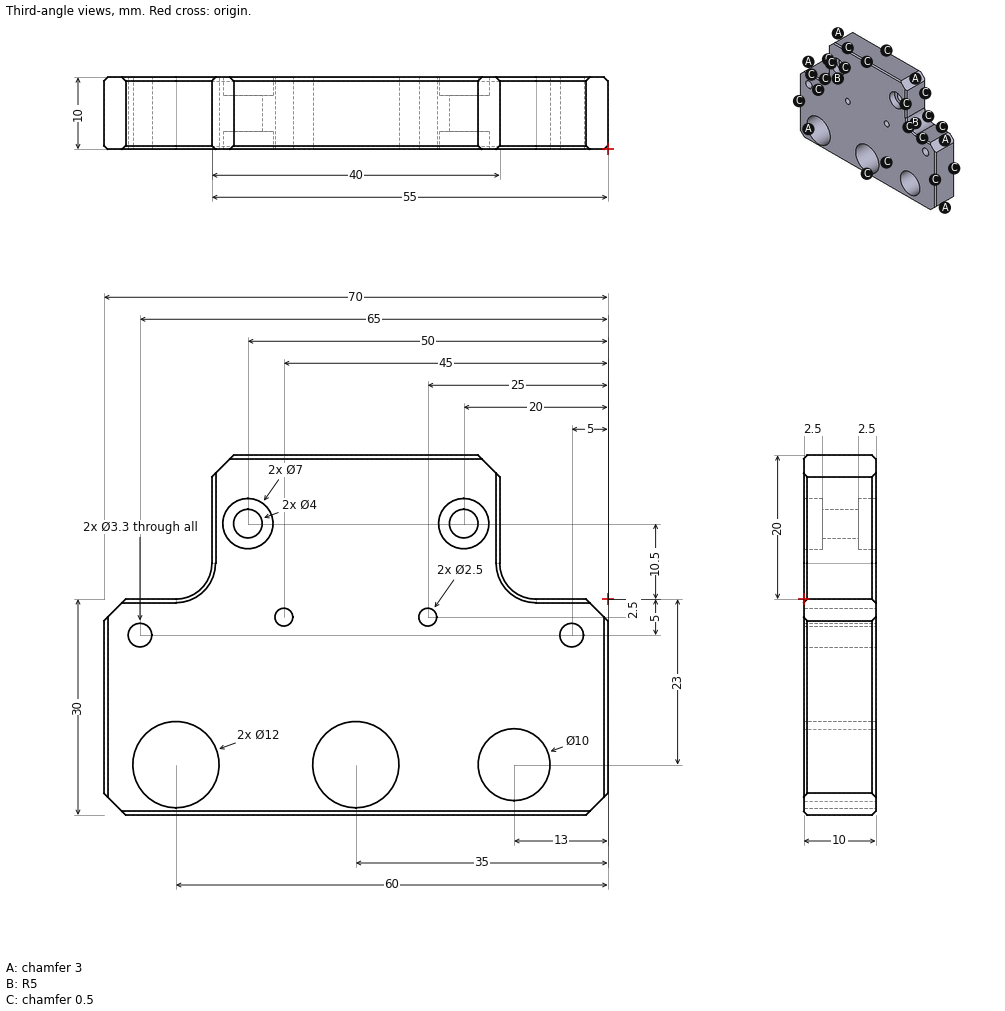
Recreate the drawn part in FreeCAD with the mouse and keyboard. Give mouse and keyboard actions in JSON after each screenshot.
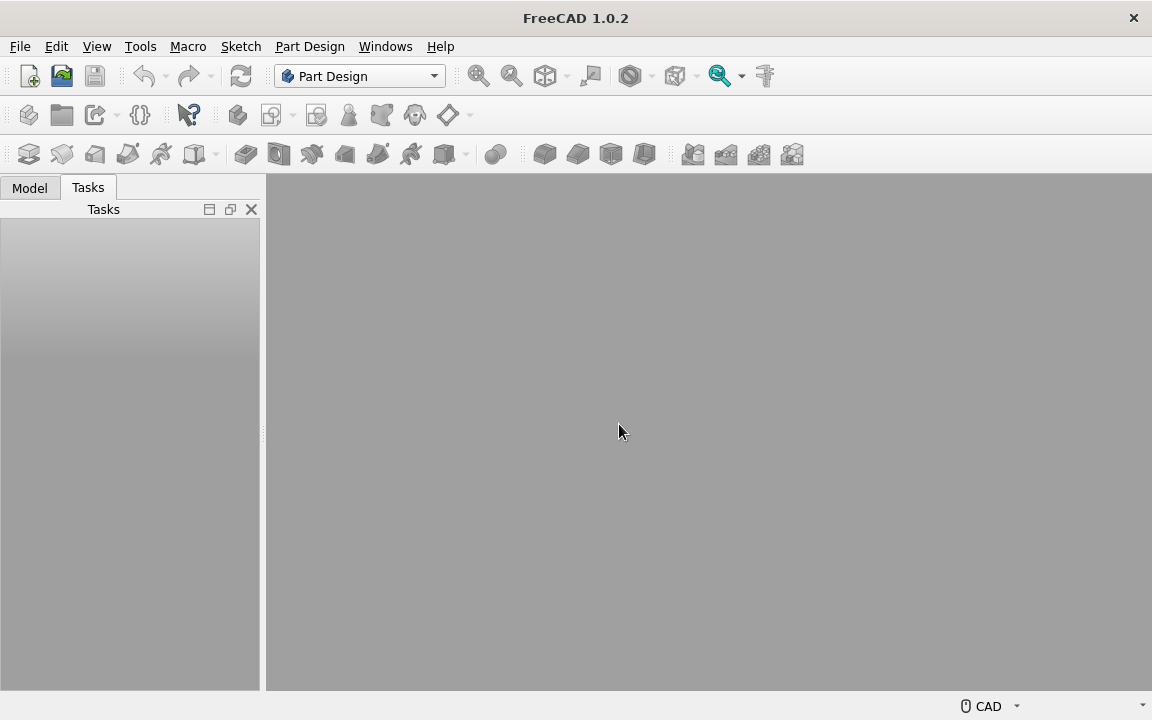
{"action": "left_click", "coordinate": [29, 76]}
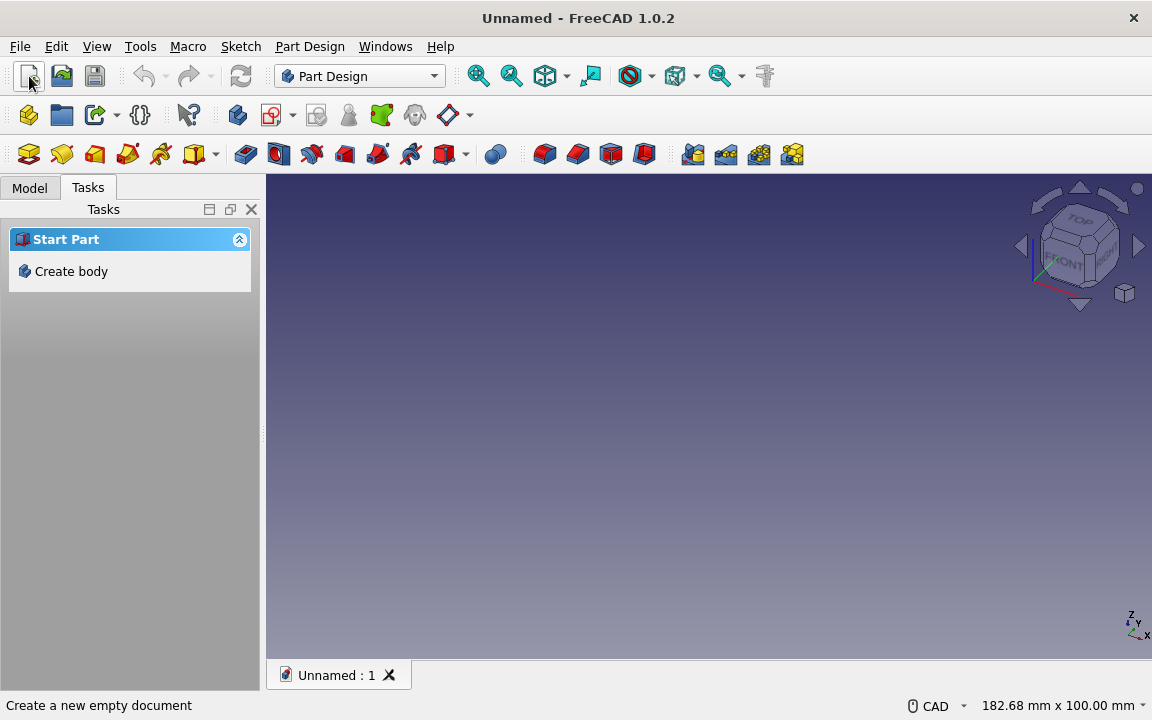
{"action": "left_click", "coordinate": [270, 116]}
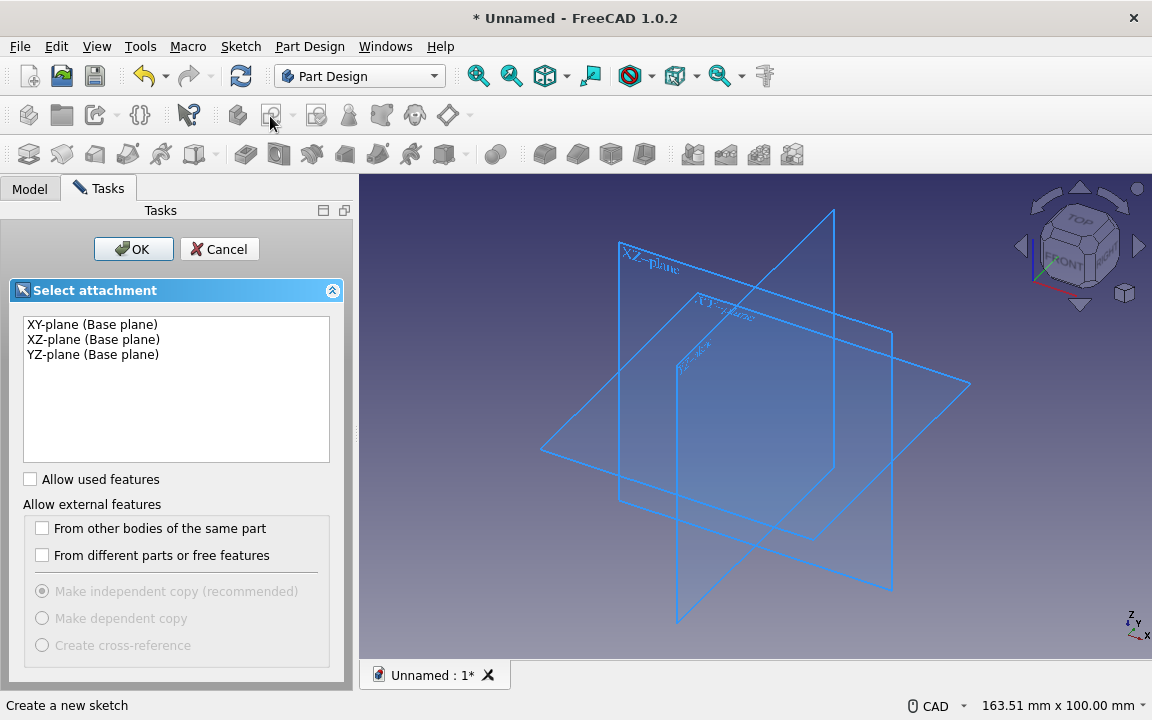
{"action": "left_click", "coordinate": [84, 340]}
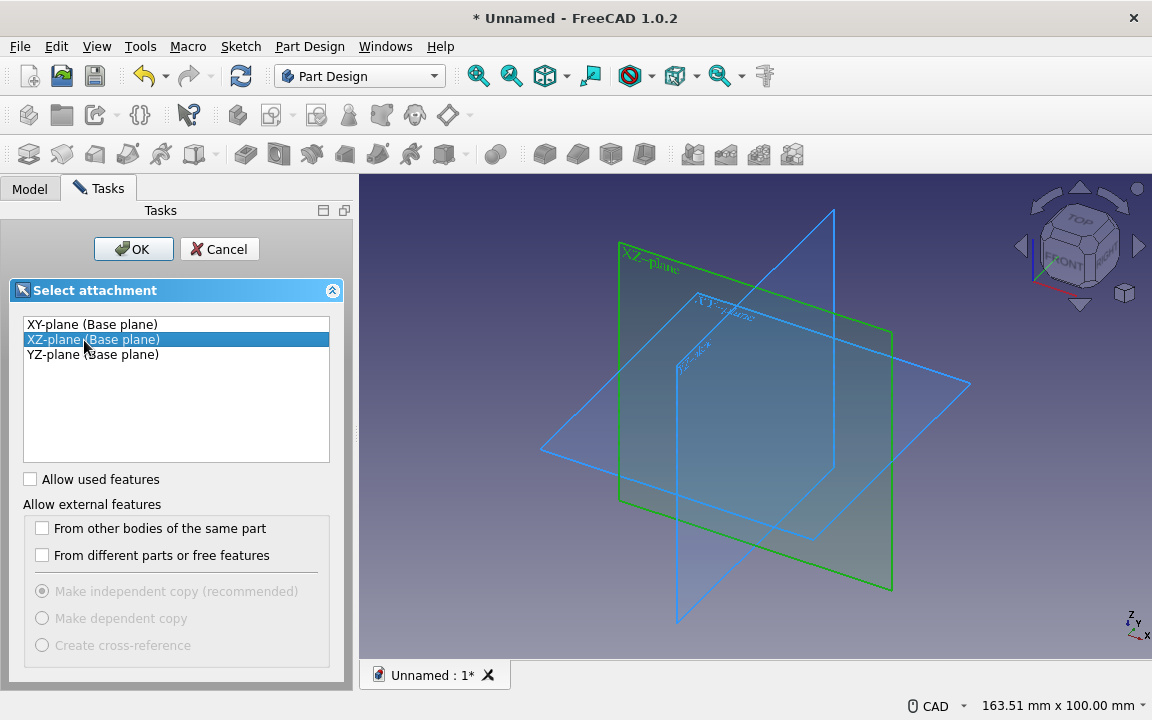
{"action": "left_click", "coordinate": [134, 249]}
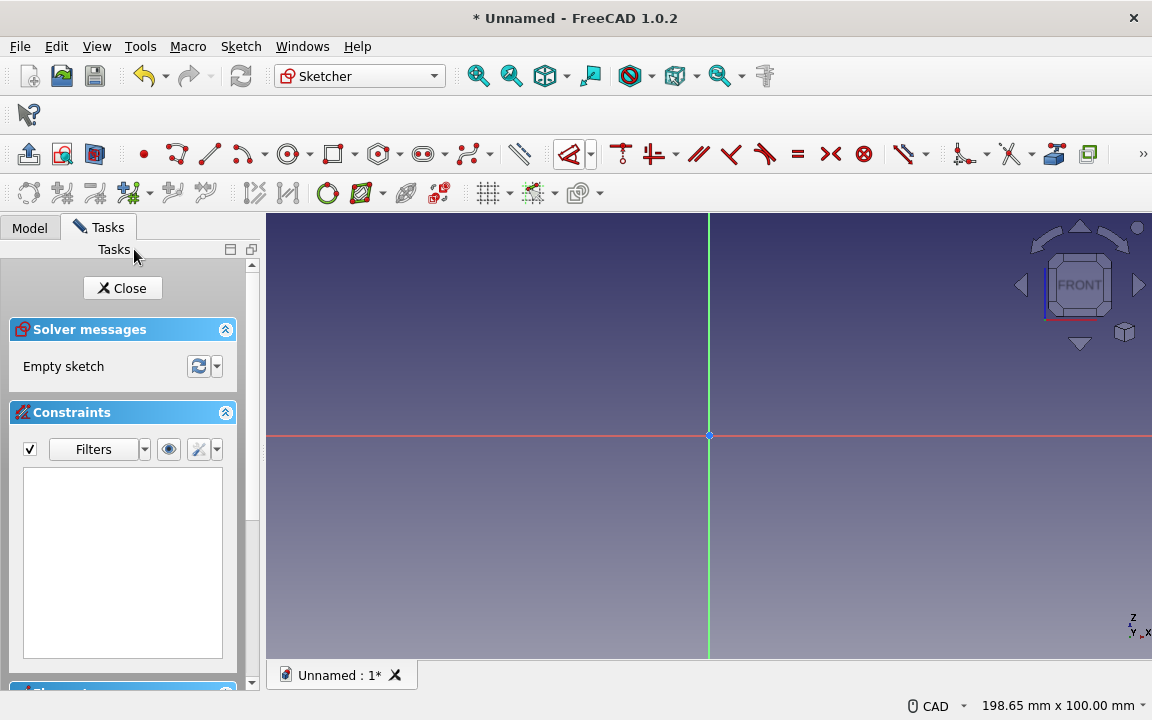
{"action": "scroll", "coordinate": [375, 631], "scroll_direction": "up", "scroll_amount": 2}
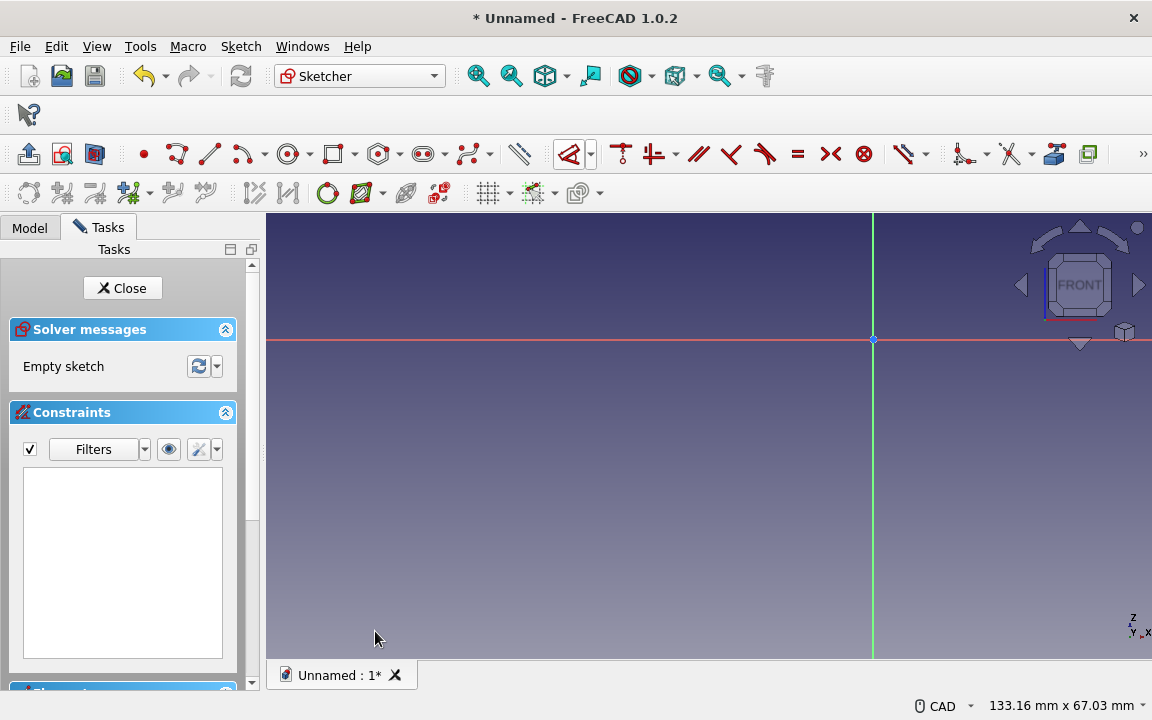
{"action": "left_click", "coordinate": [332, 154]}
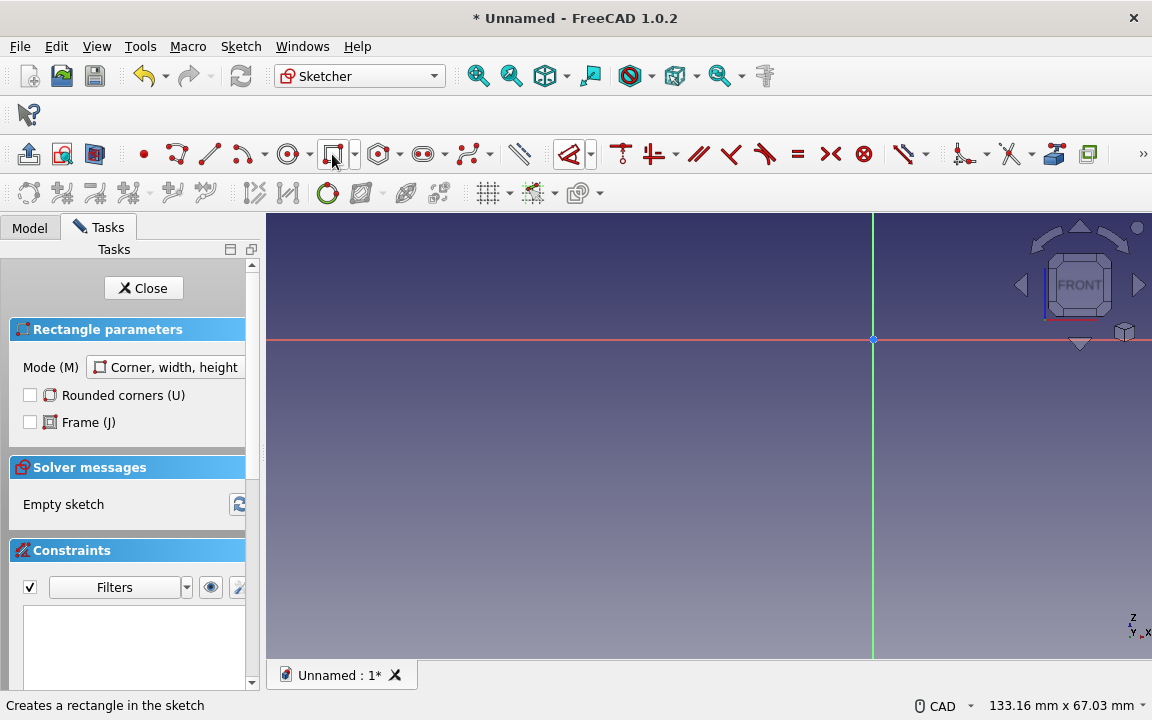
{"action": "left_click", "coordinate": [873, 340]}
{"action": "left_click", "coordinate": [407, 539]}
{"action": "key", "text": "Escape"}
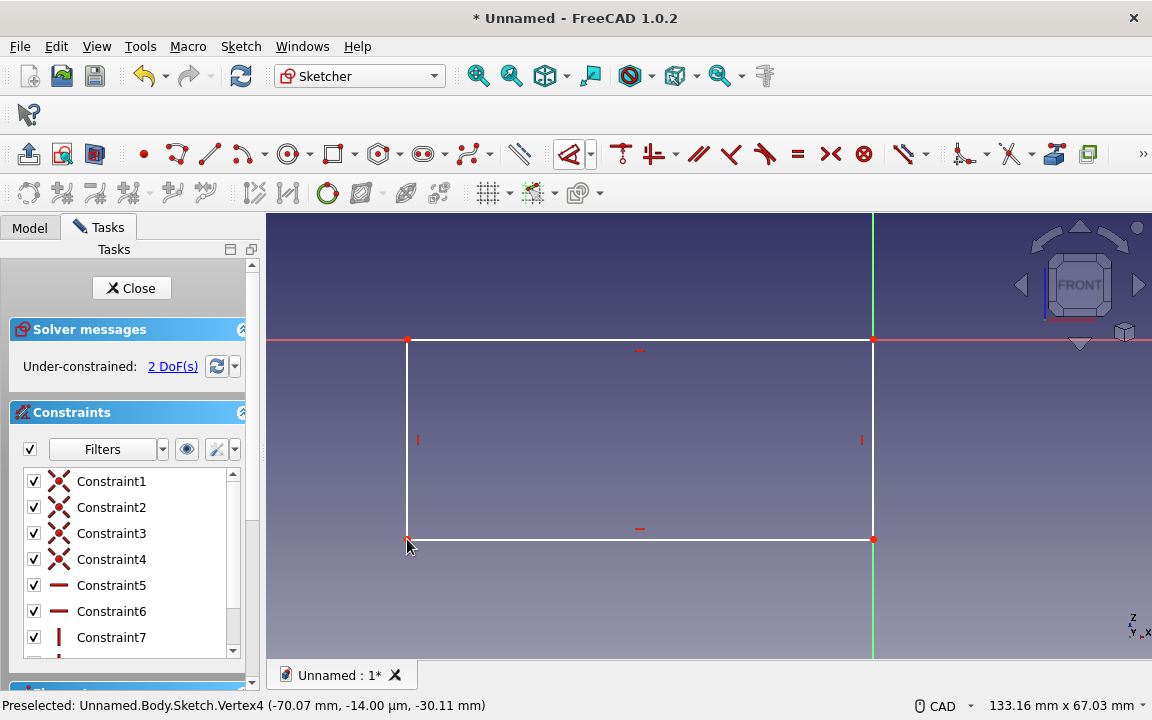
{"action": "left_click", "coordinate": [733, 340]}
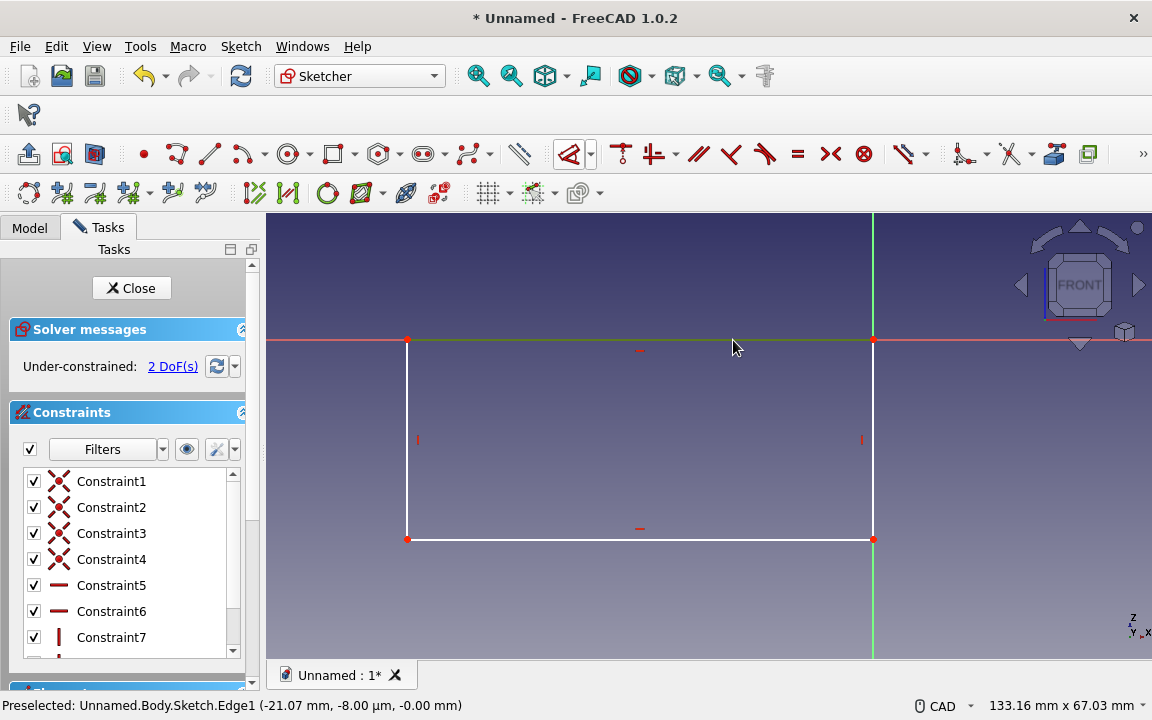
{"action": "key", "text": "l"}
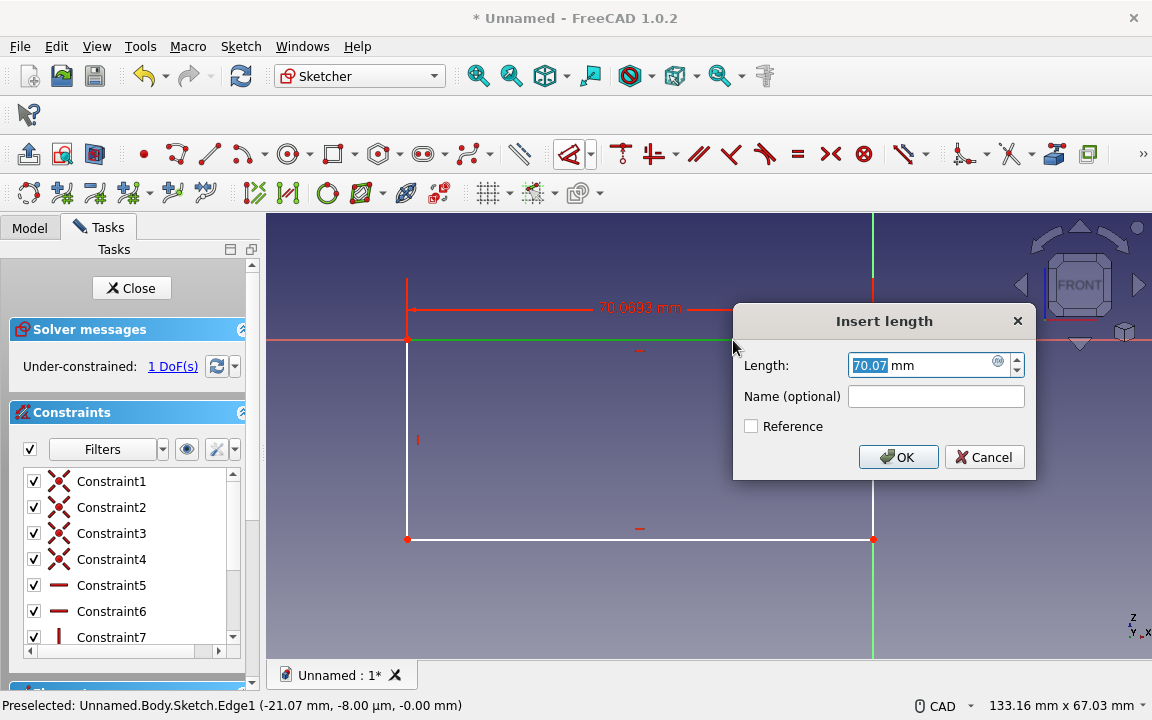
{"action": "type", "text": "70"}
{"action": "key", "text": "Return"}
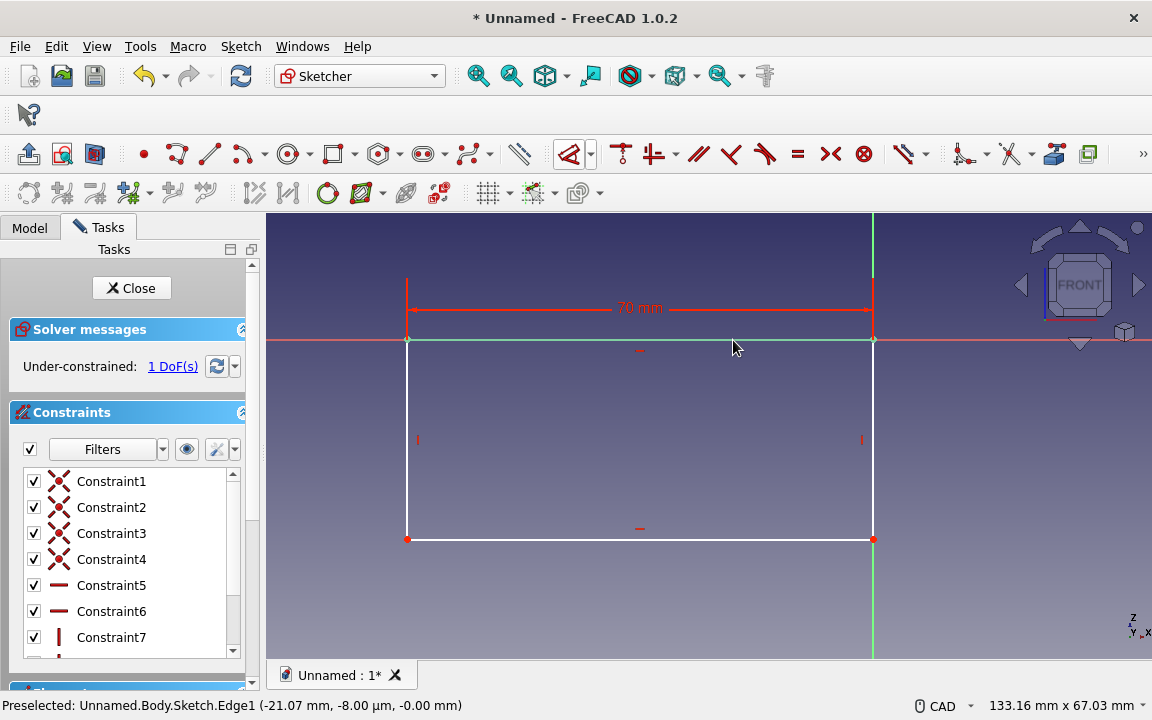
{"action": "left_click", "coordinate": [407, 400]}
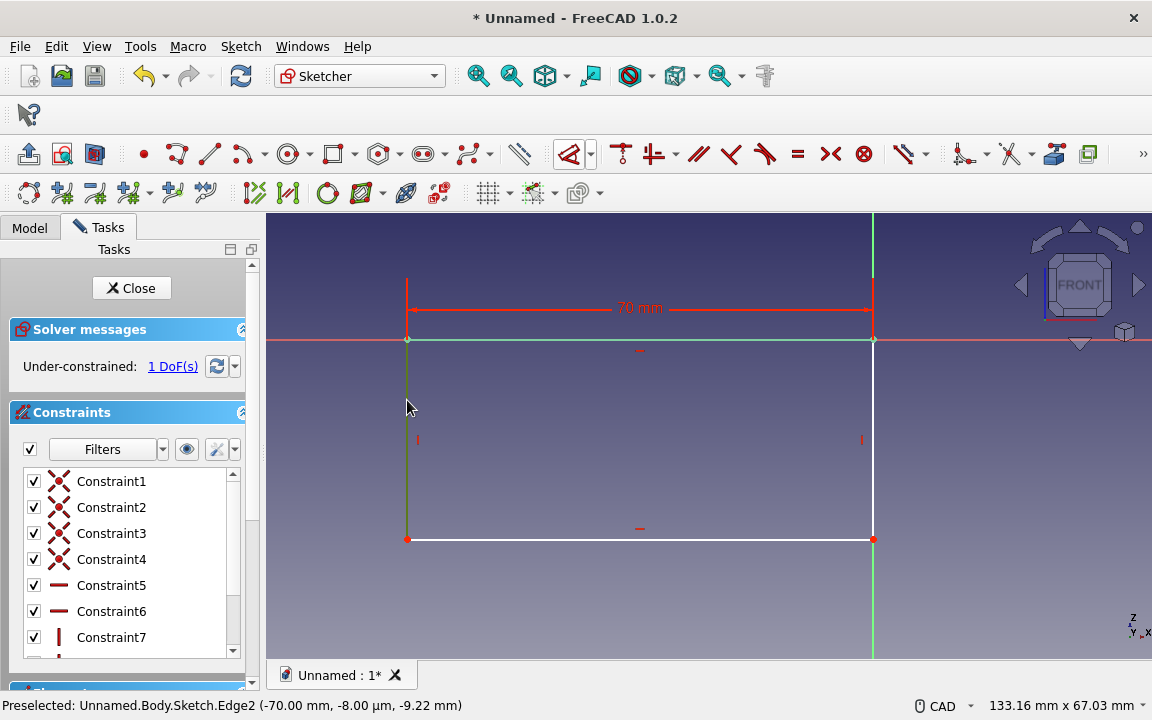
{"action": "left_click", "coordinate": [590, 154]}